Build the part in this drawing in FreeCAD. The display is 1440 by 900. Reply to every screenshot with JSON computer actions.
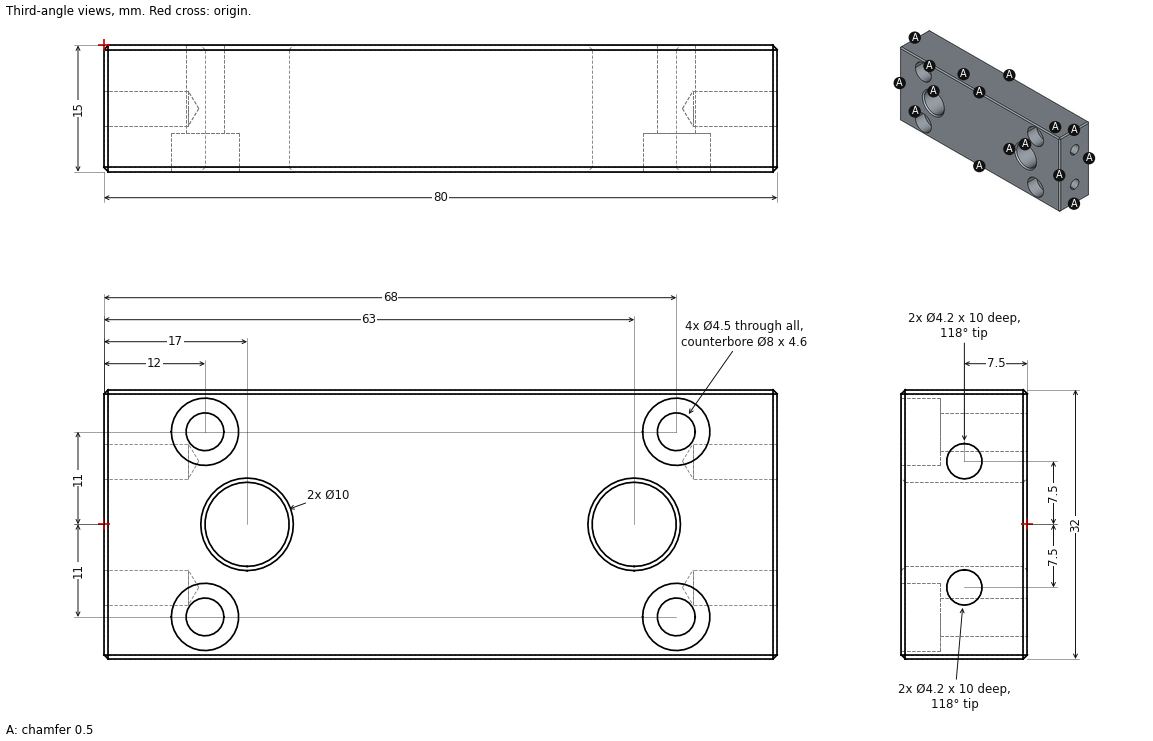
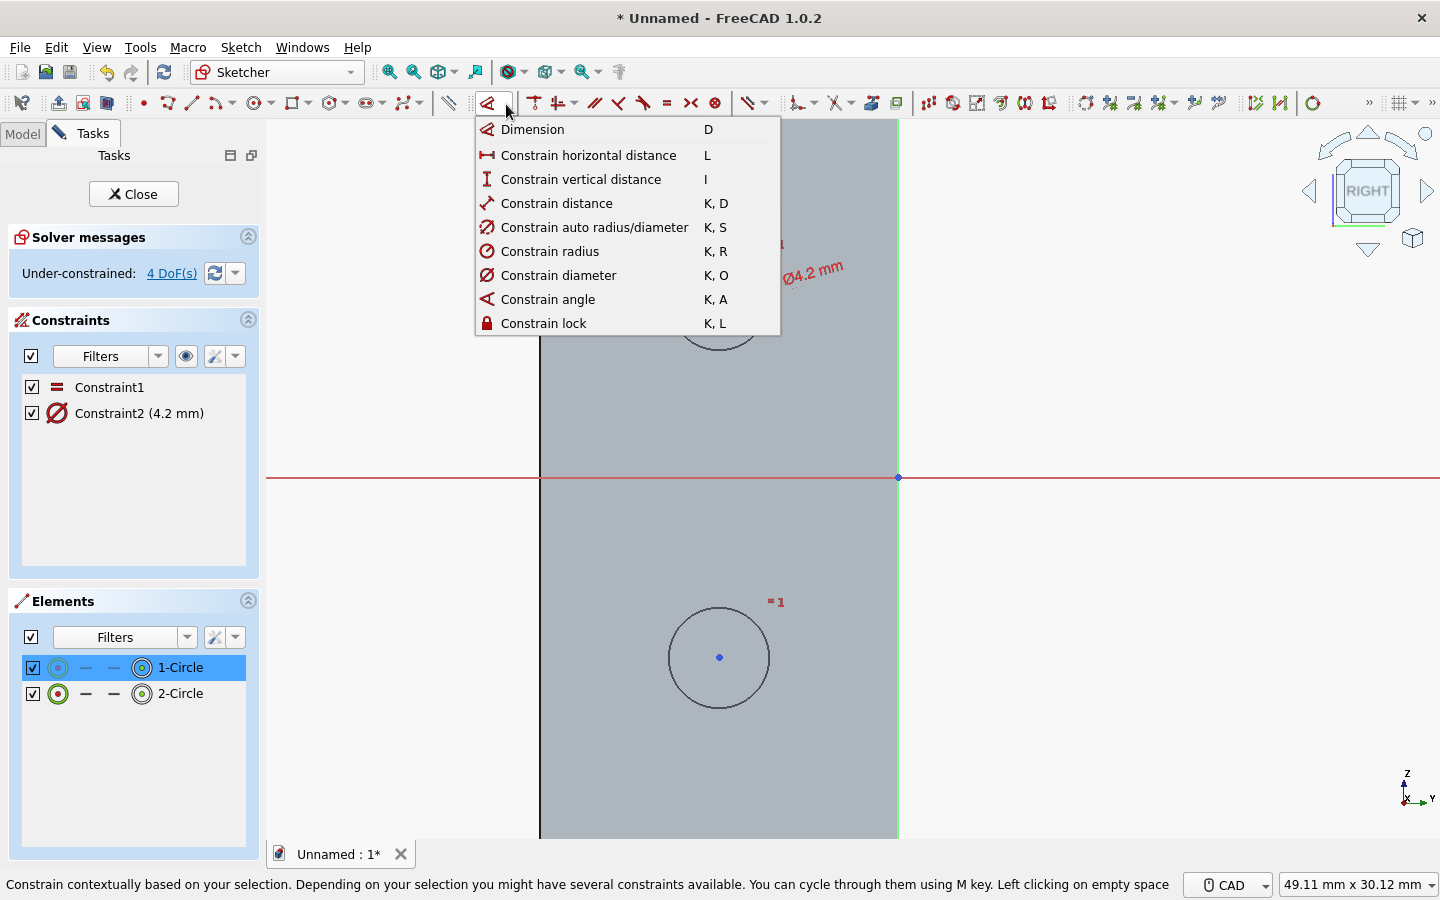
{"action": "left_click", "coordinate": [628, 155]}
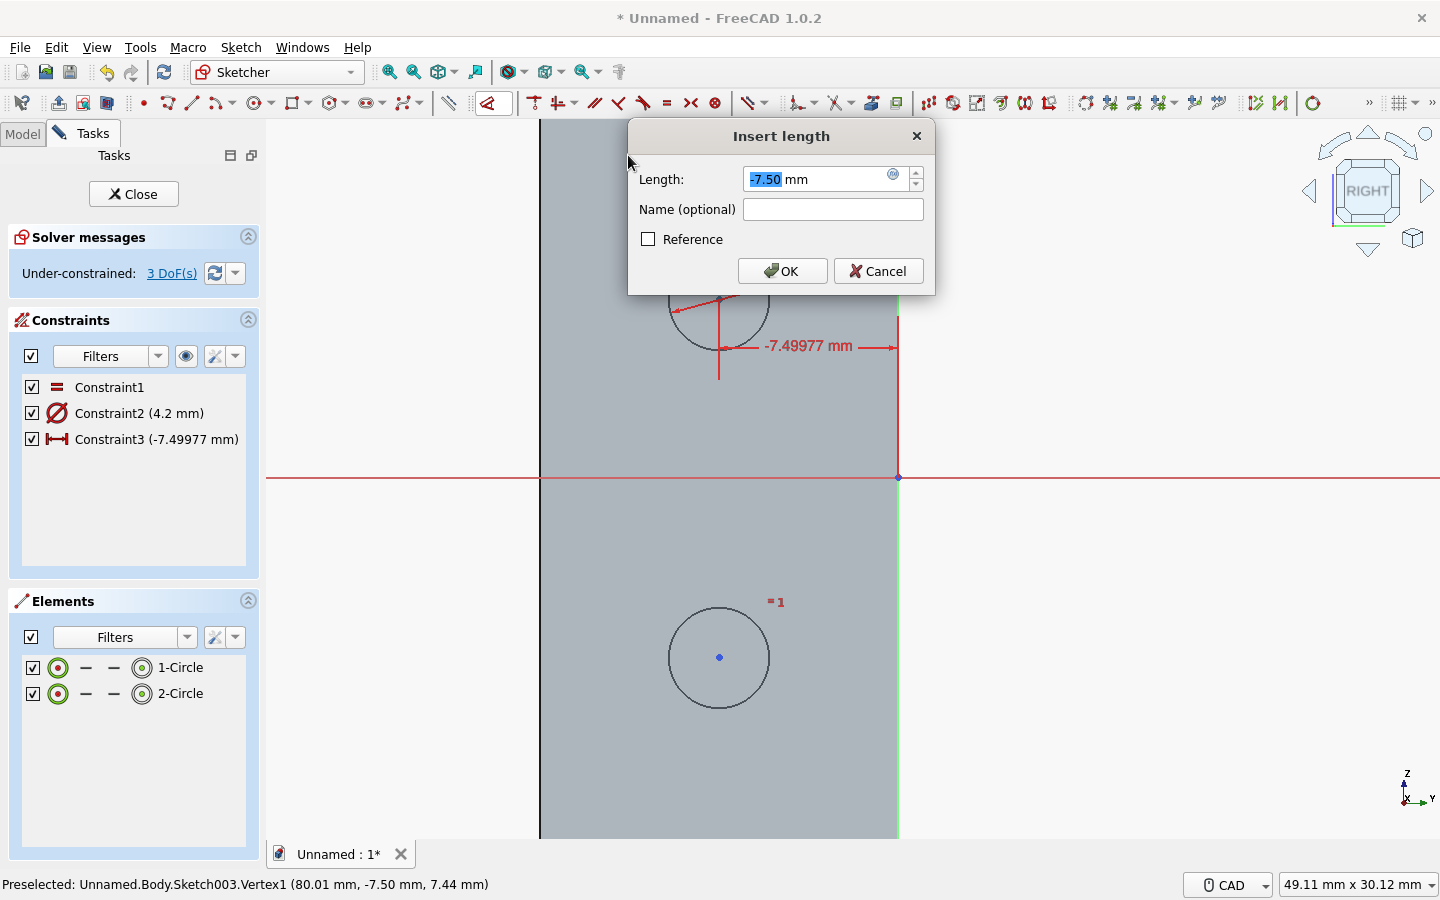
{"action": "type", "text": "-7.5"}
{"action": "key", "text": "Return"}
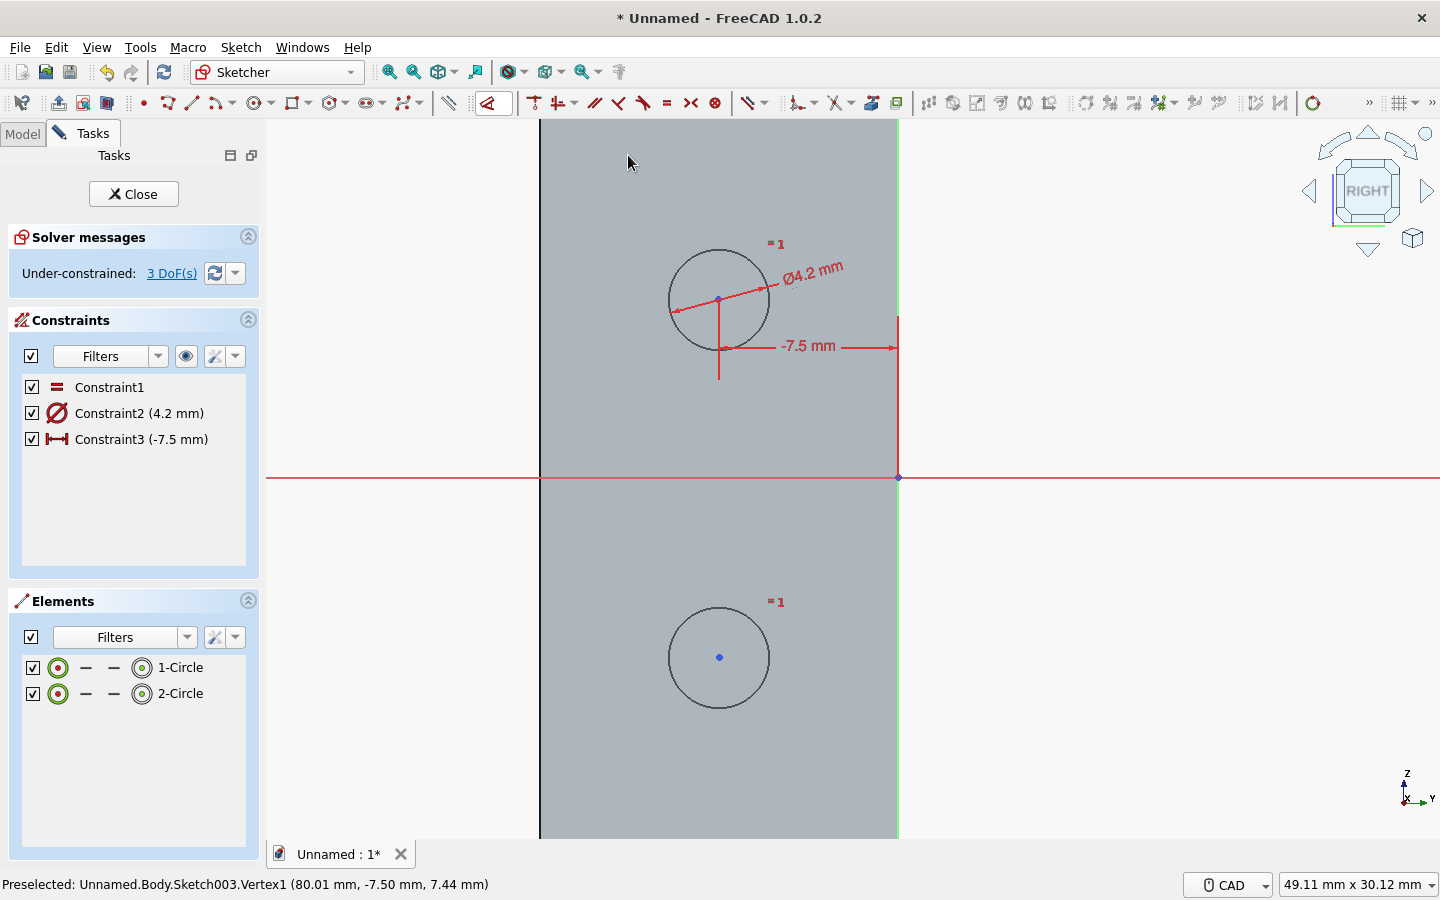
{"action": "left_click", "coordinate": [719, 300]}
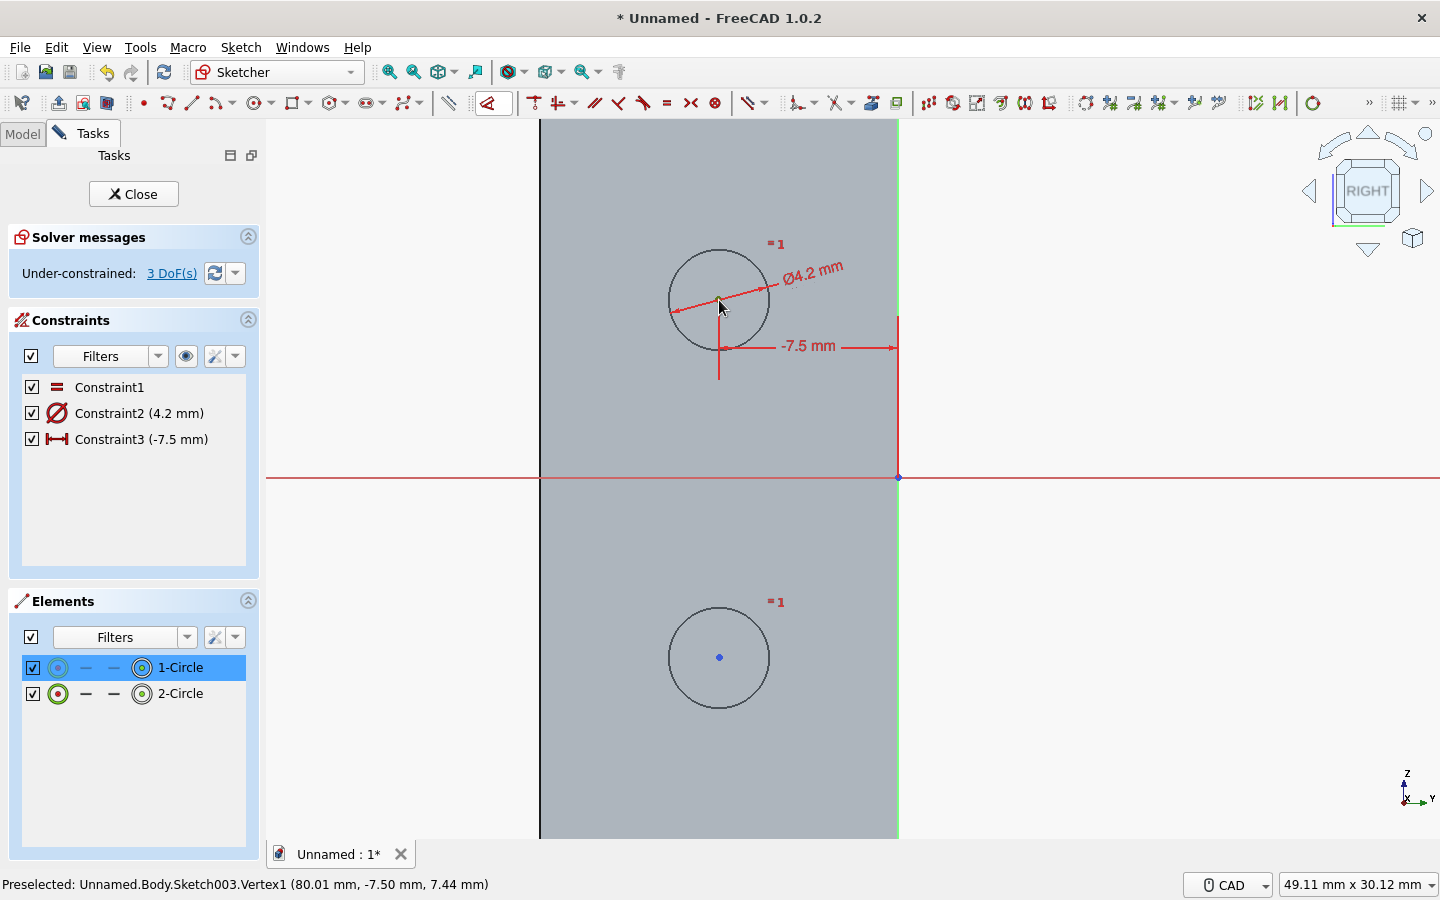
{"action": "left_click", "coordinate": [506, 104]}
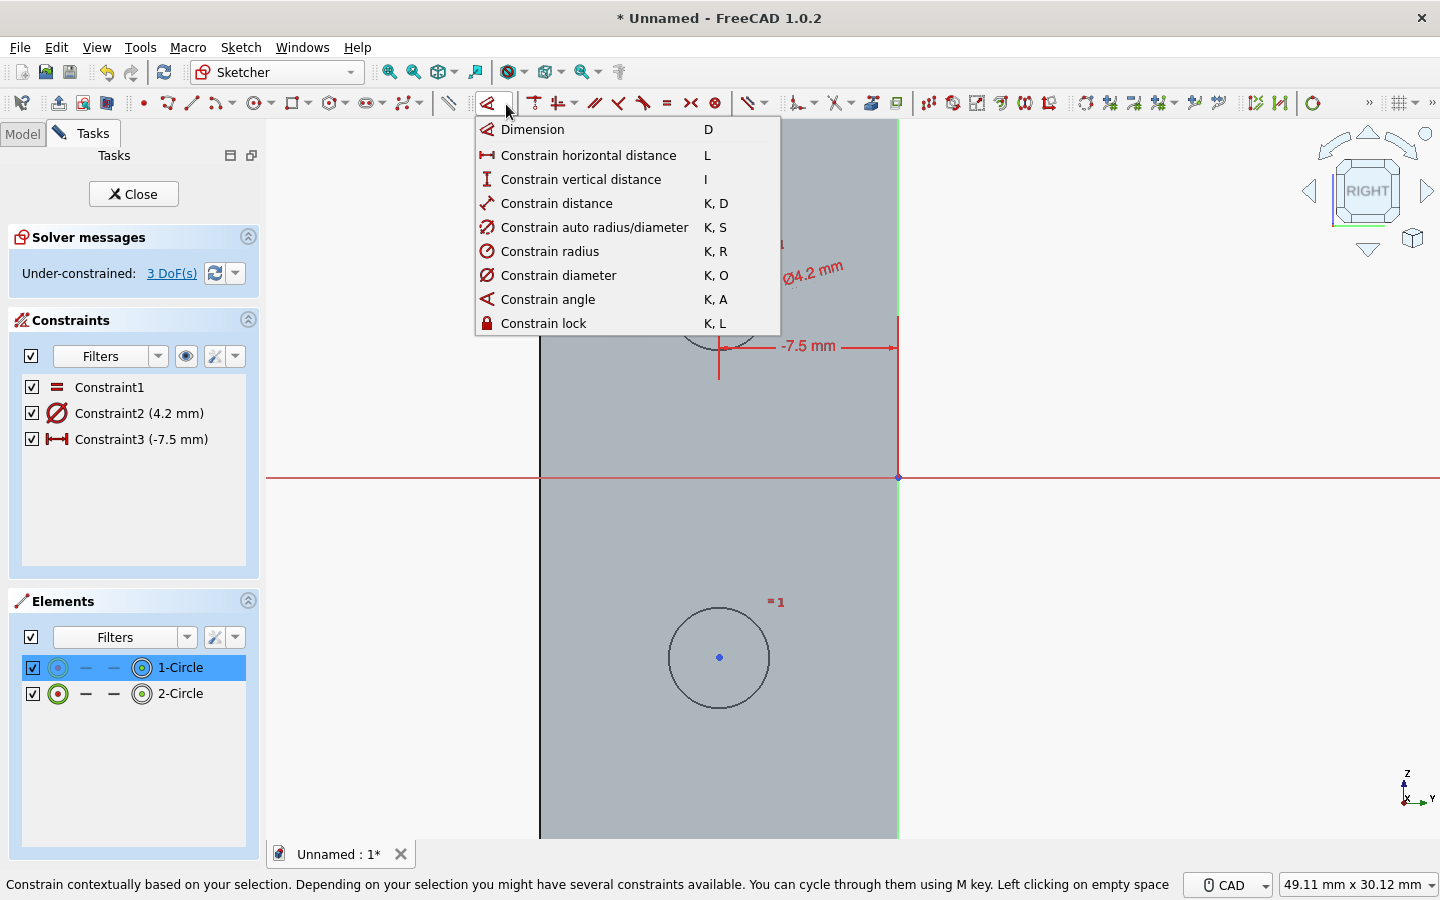
{"action": "left_click", "coordinate": [628, 179]}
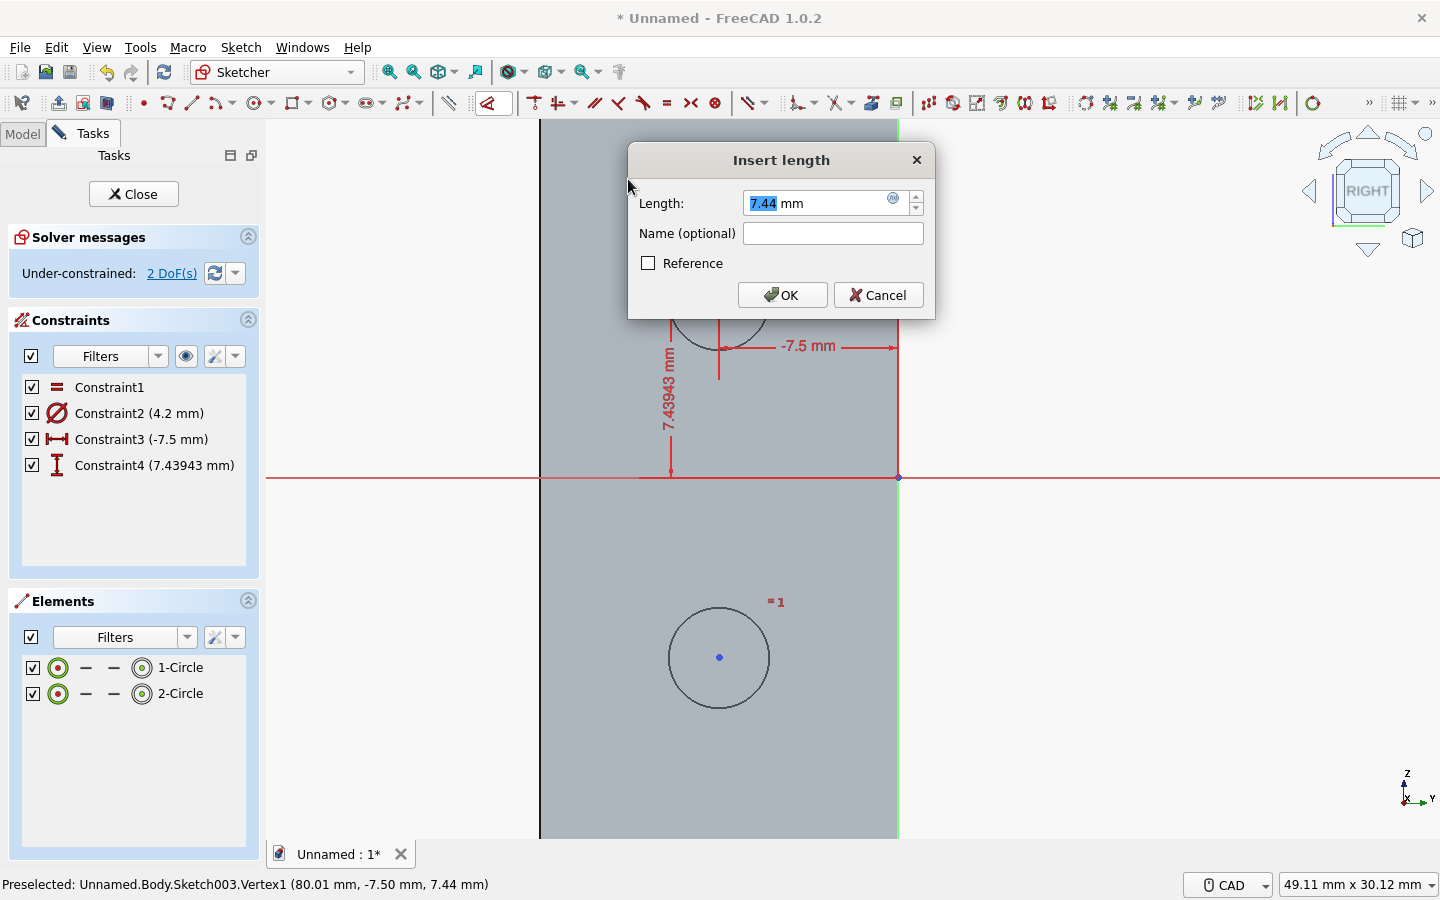
{"action": "type", "text": "7.5"}
{"action": "key", "text": "Return"}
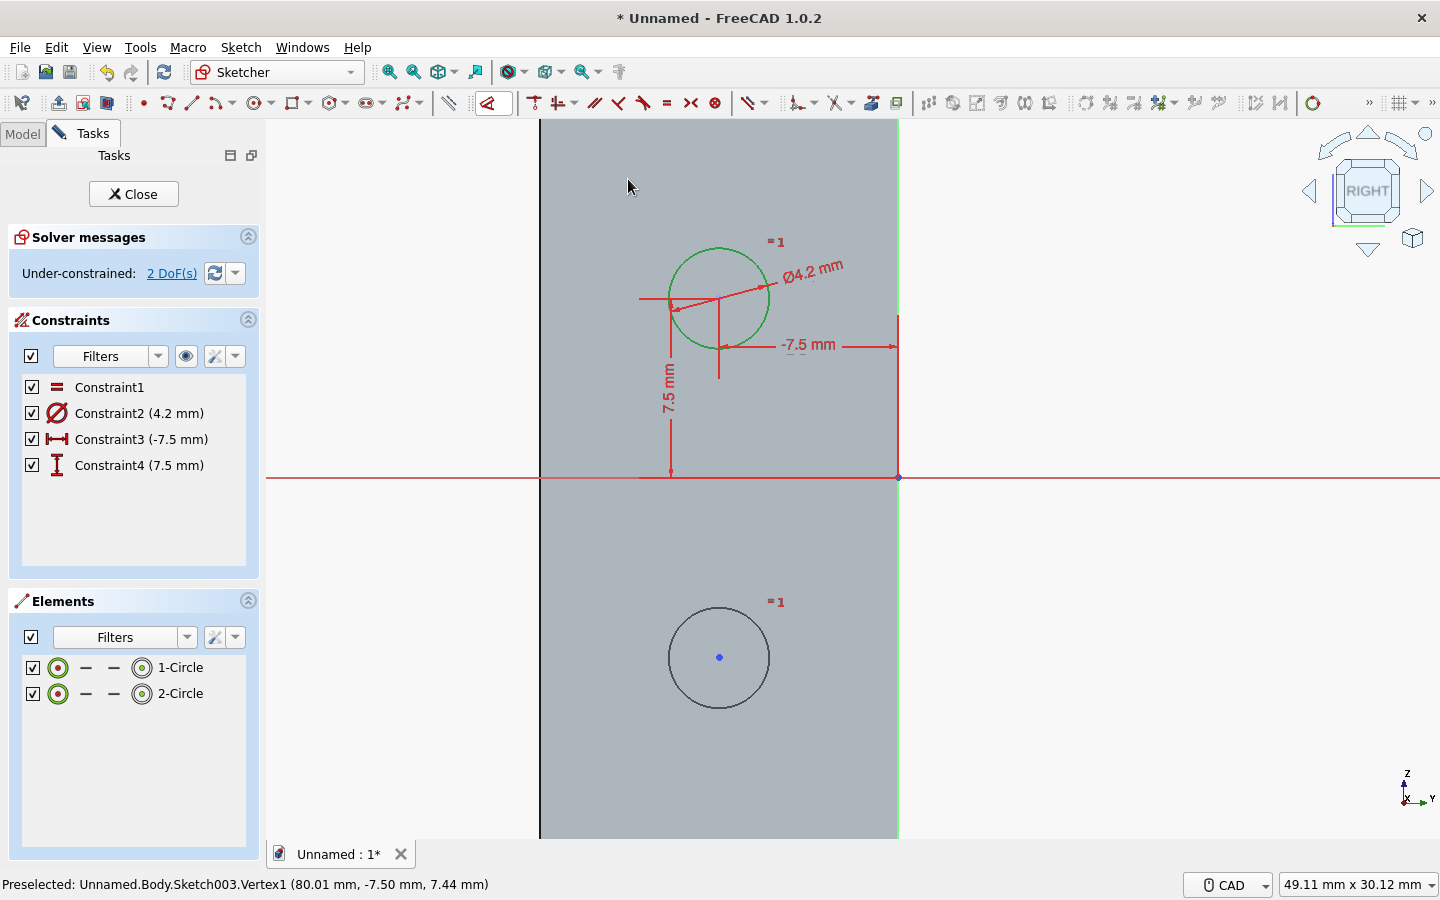
{"action": "left_click", "coordinate": [719, 658]}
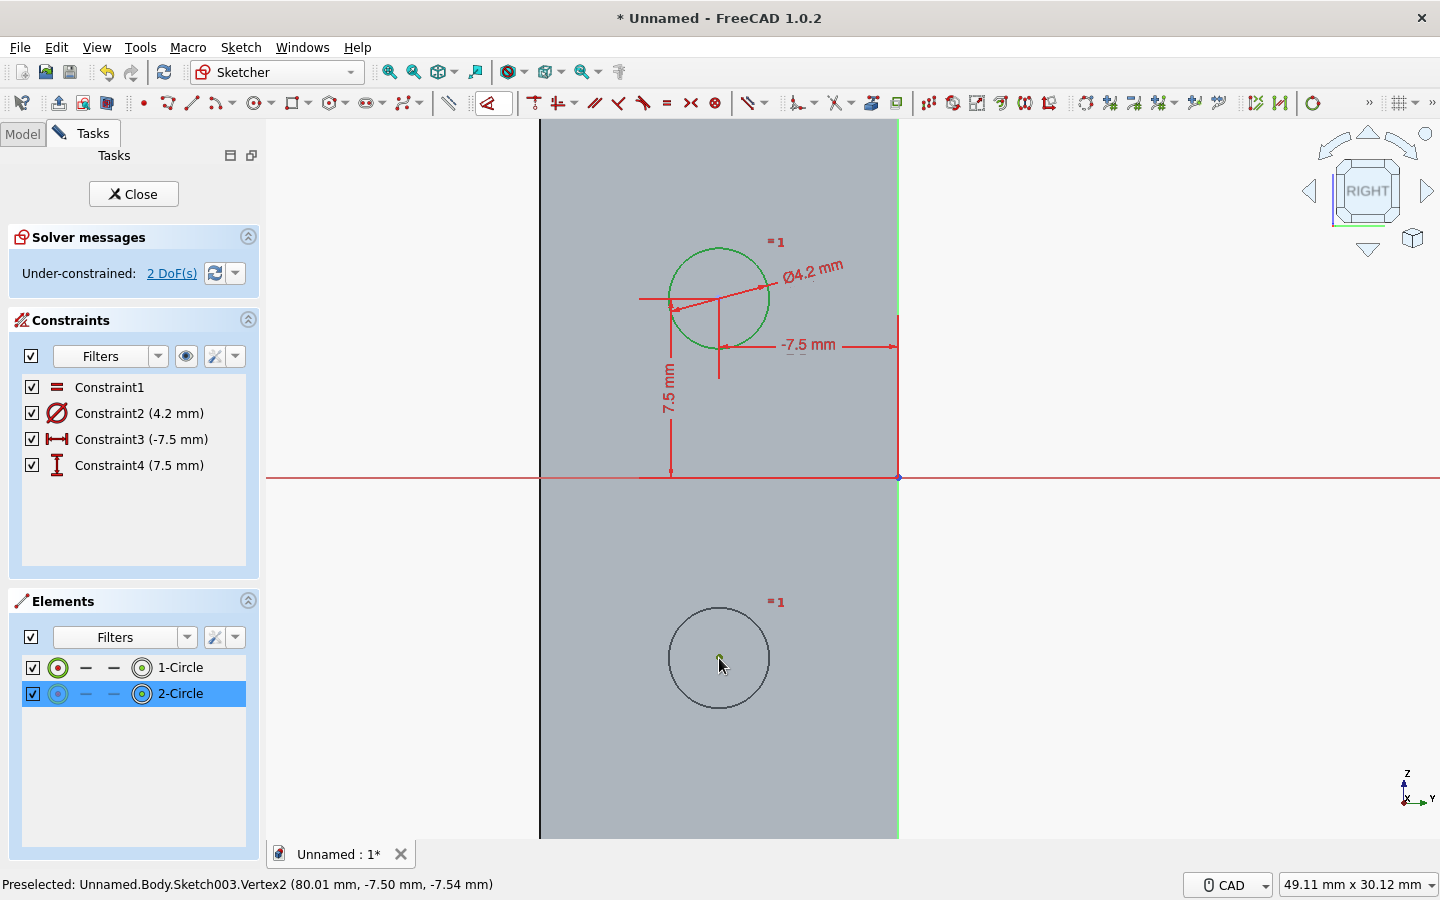
{"action": "key", "text": "l"}